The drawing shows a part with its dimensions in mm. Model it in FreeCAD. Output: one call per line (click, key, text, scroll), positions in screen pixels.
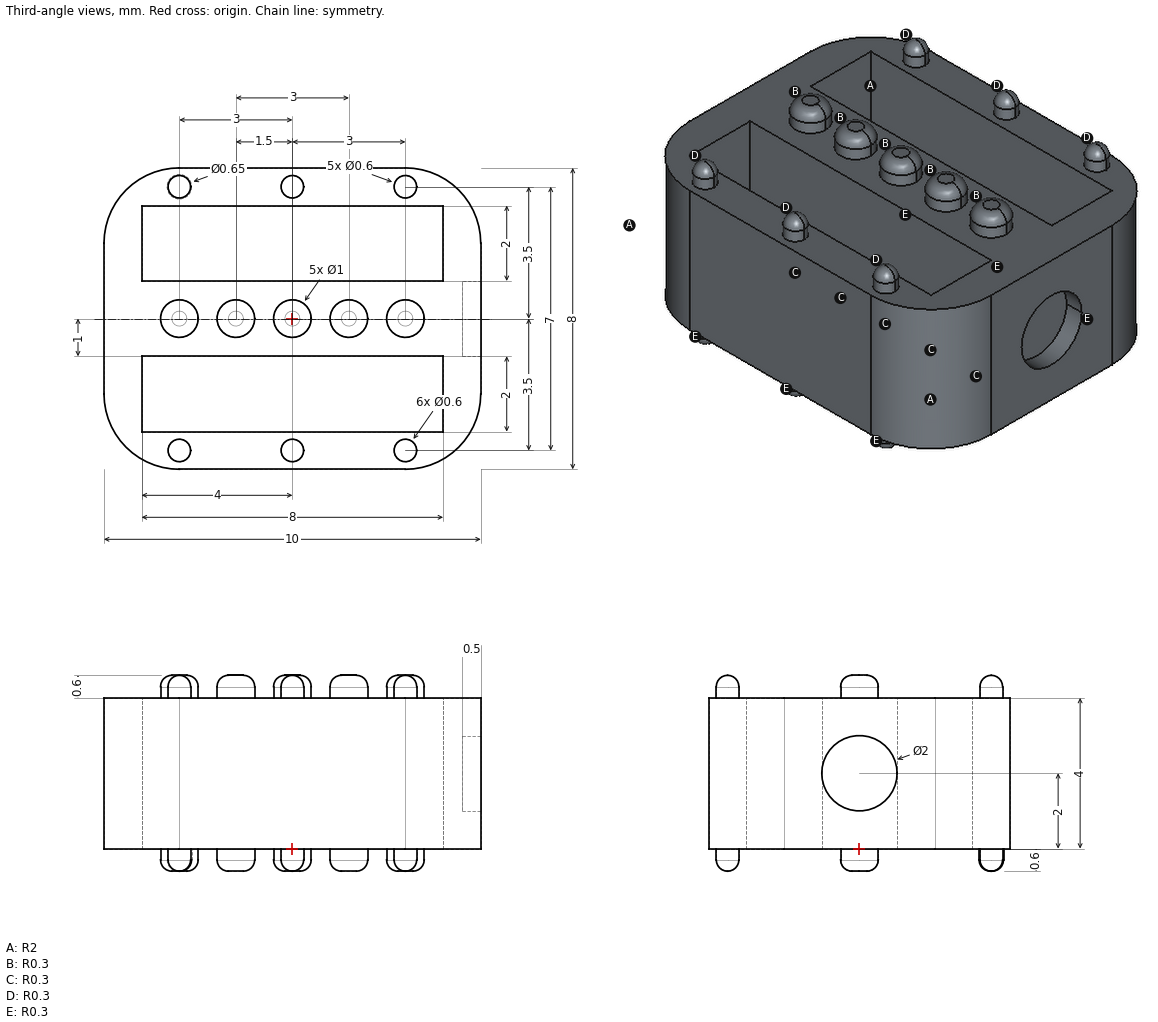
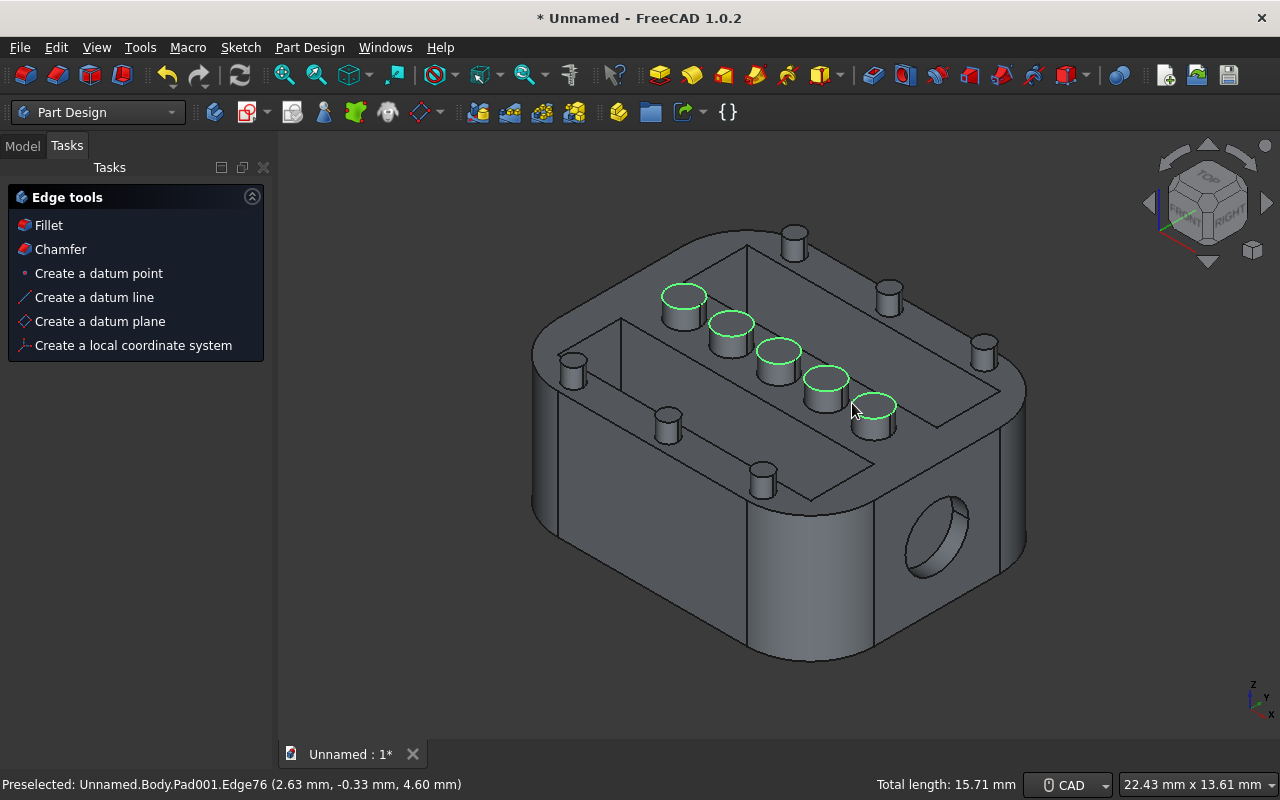
click(26, 76)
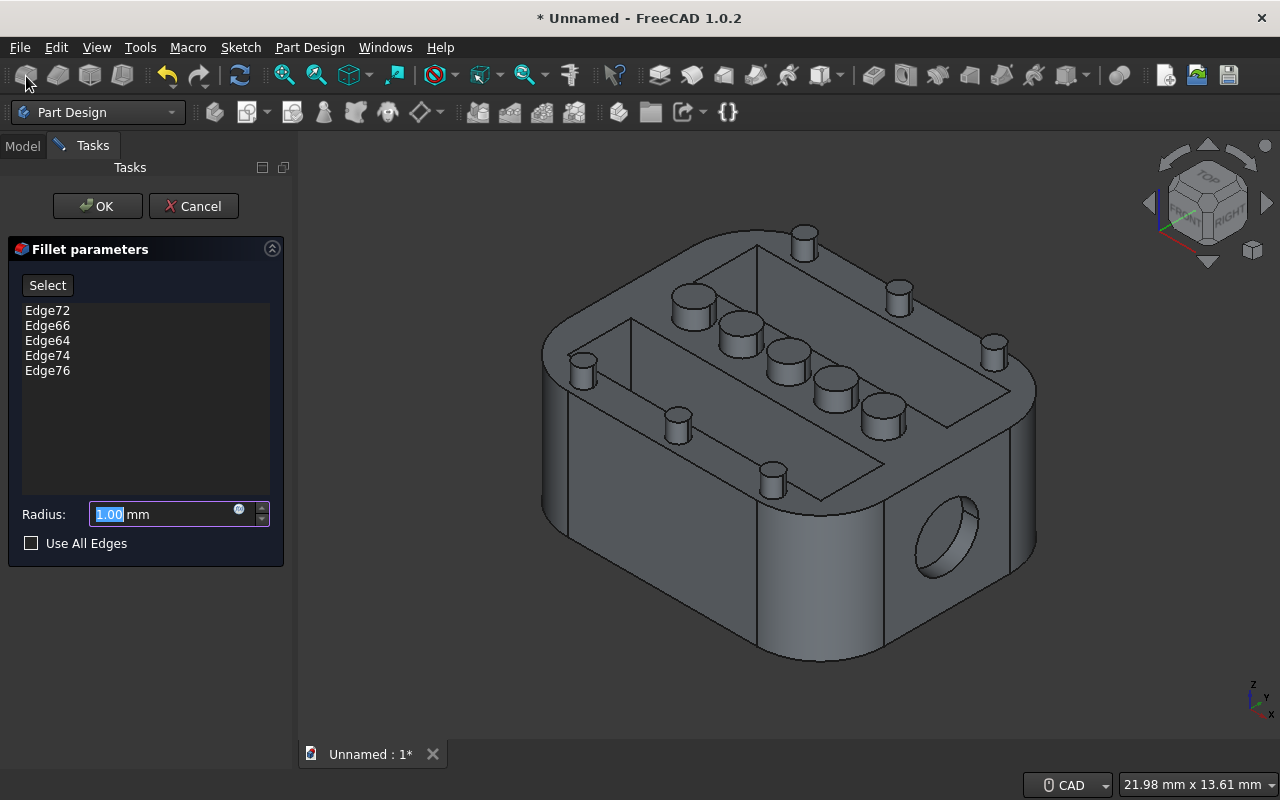
text(0.3)
key(Tab)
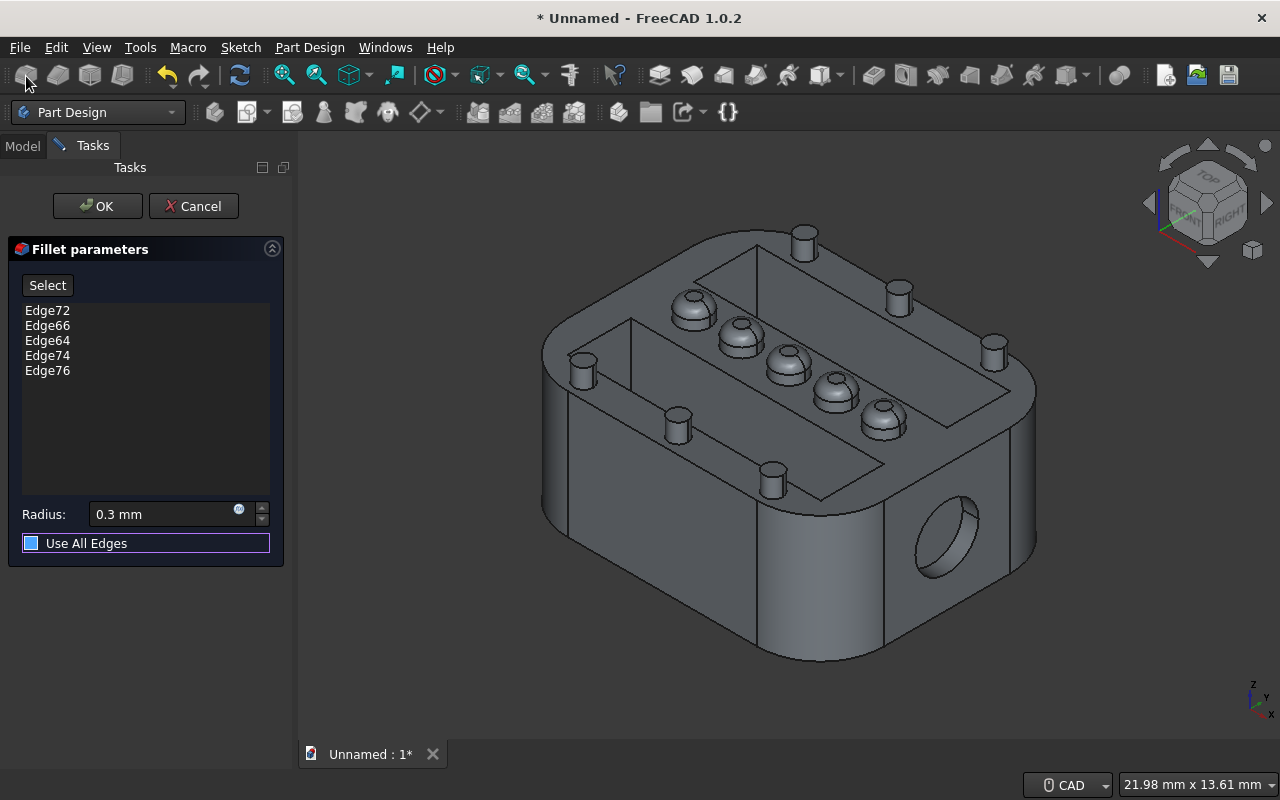
click(98, 206)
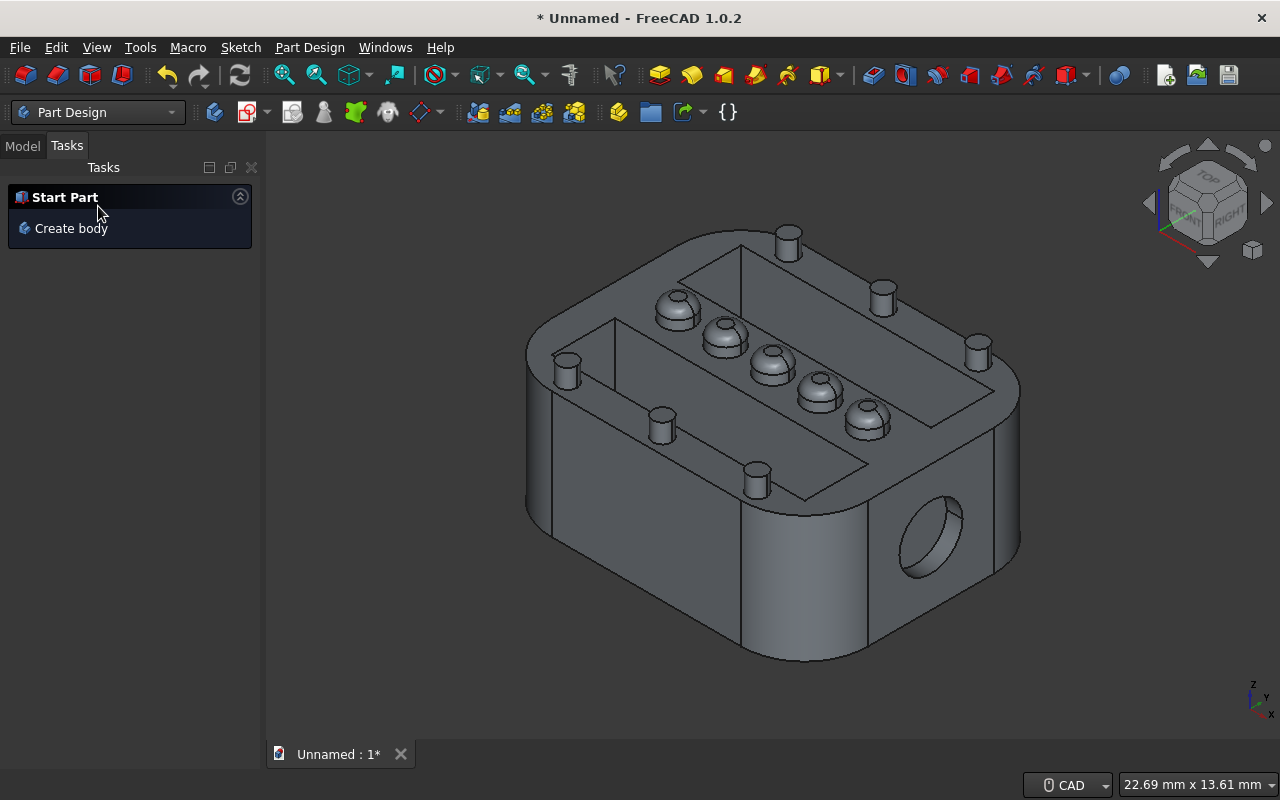
click(23, 145)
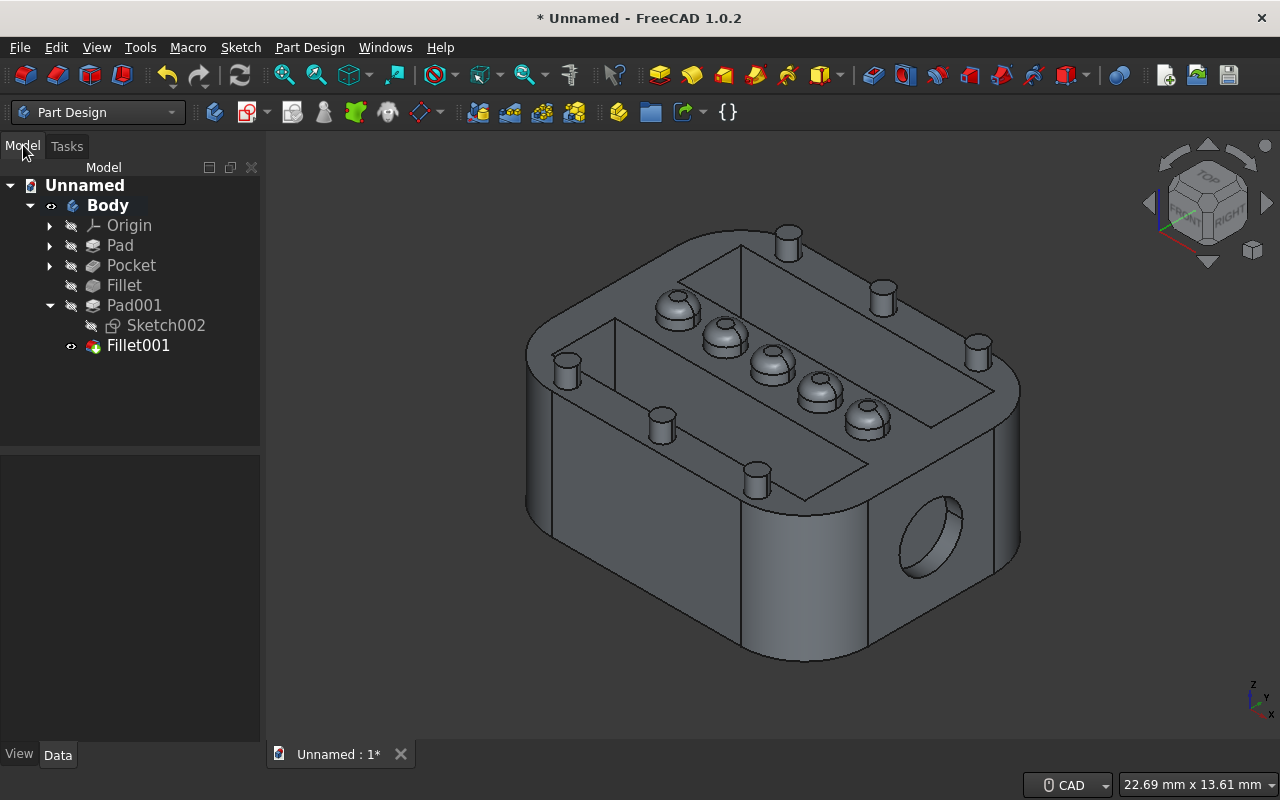
click(50, 226)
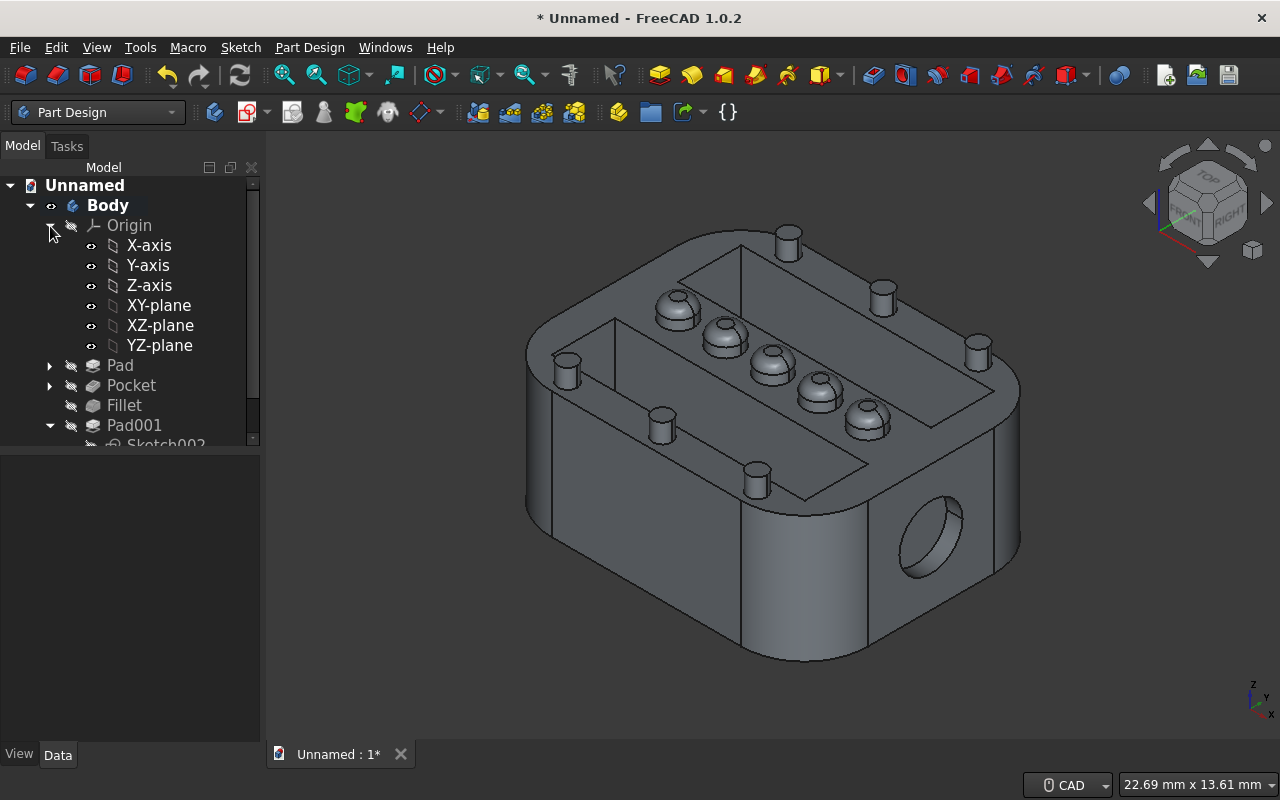
click(136, 306)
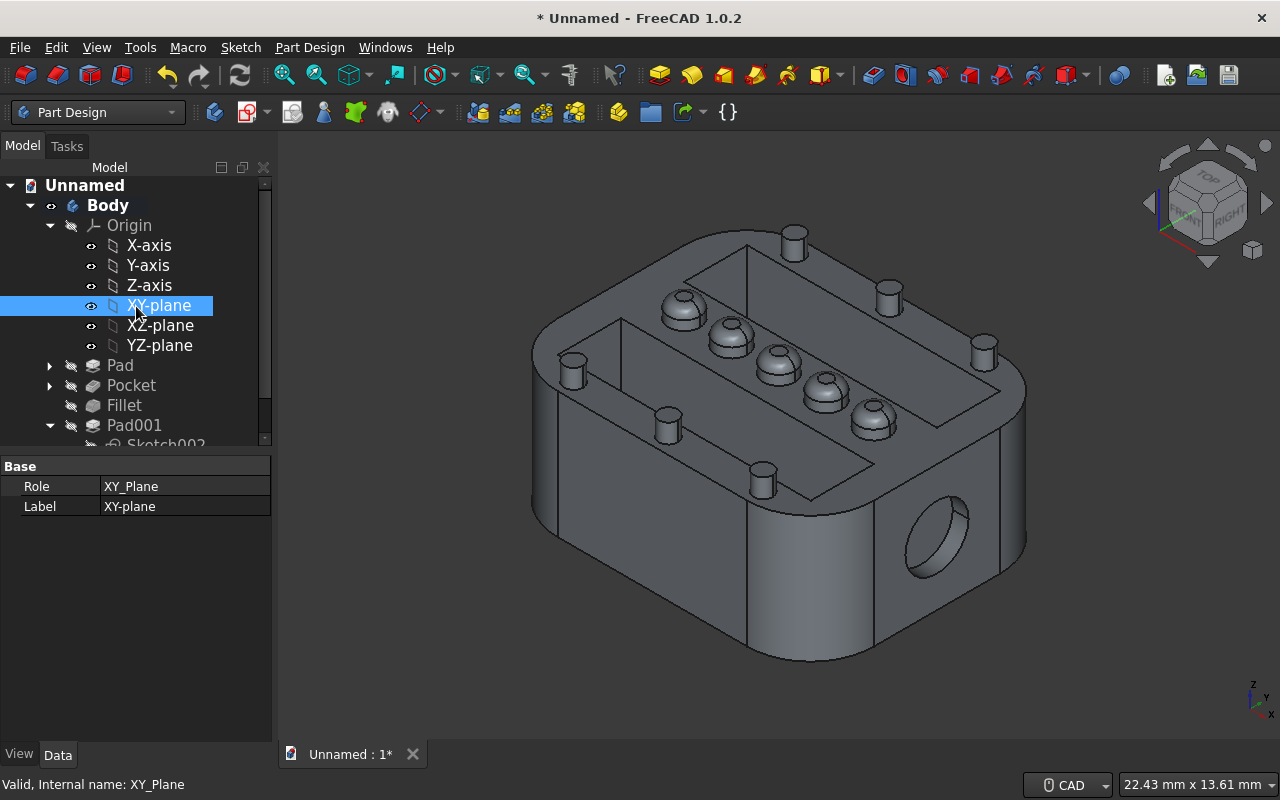
click(420, 112)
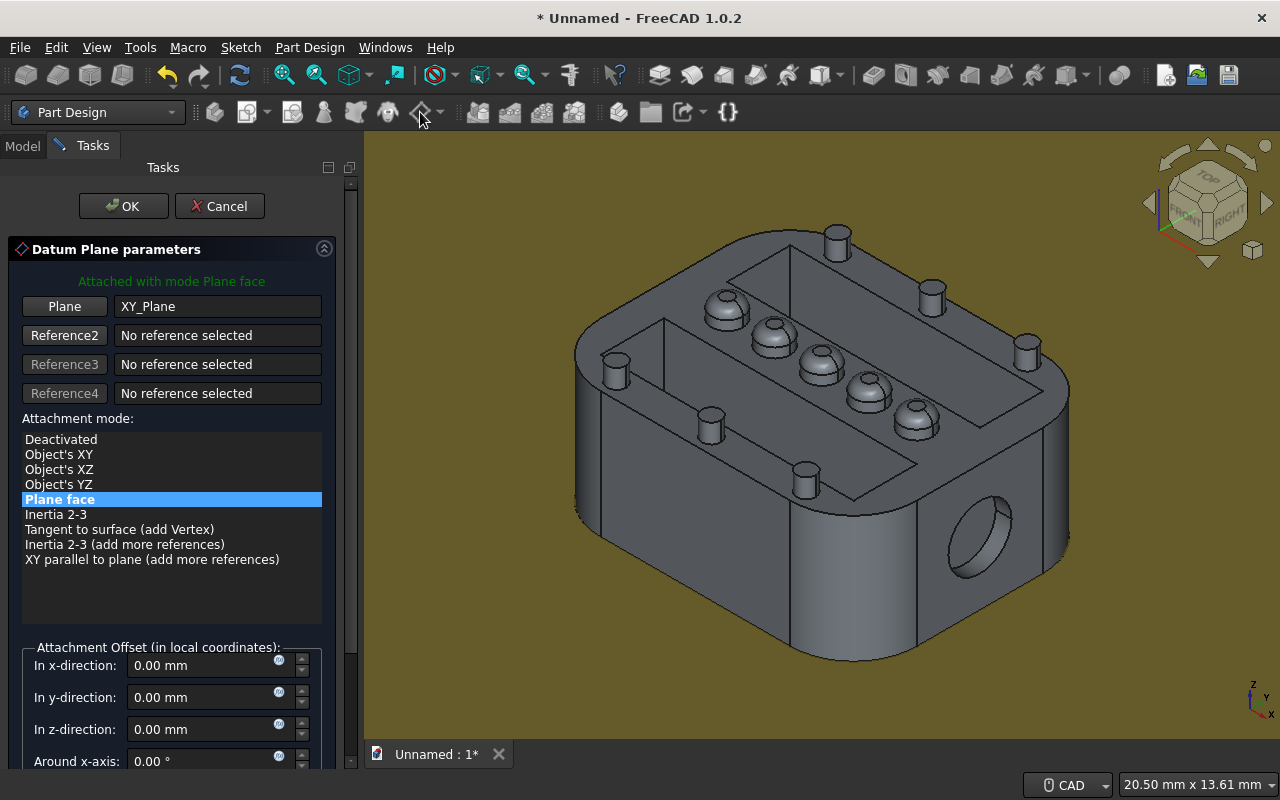
triple_click(210, 729)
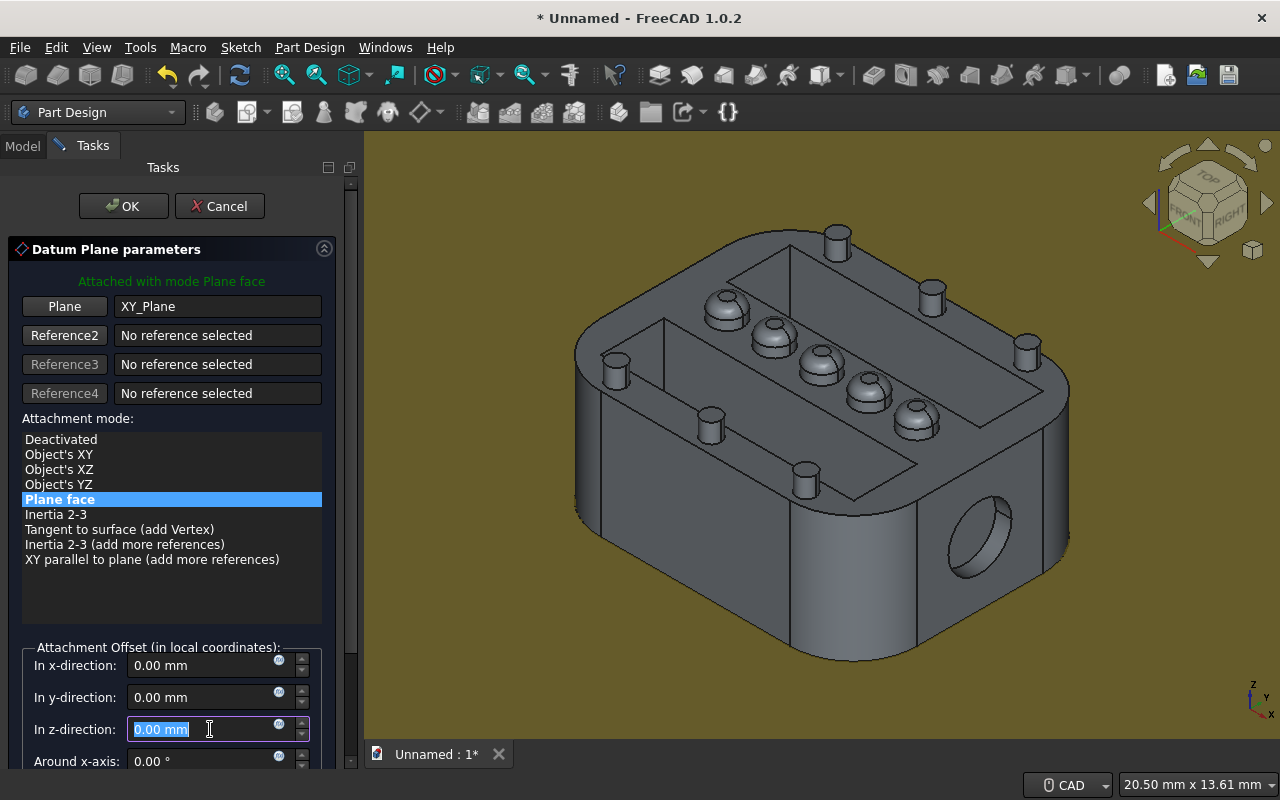
text(-0.6)
key(Tab)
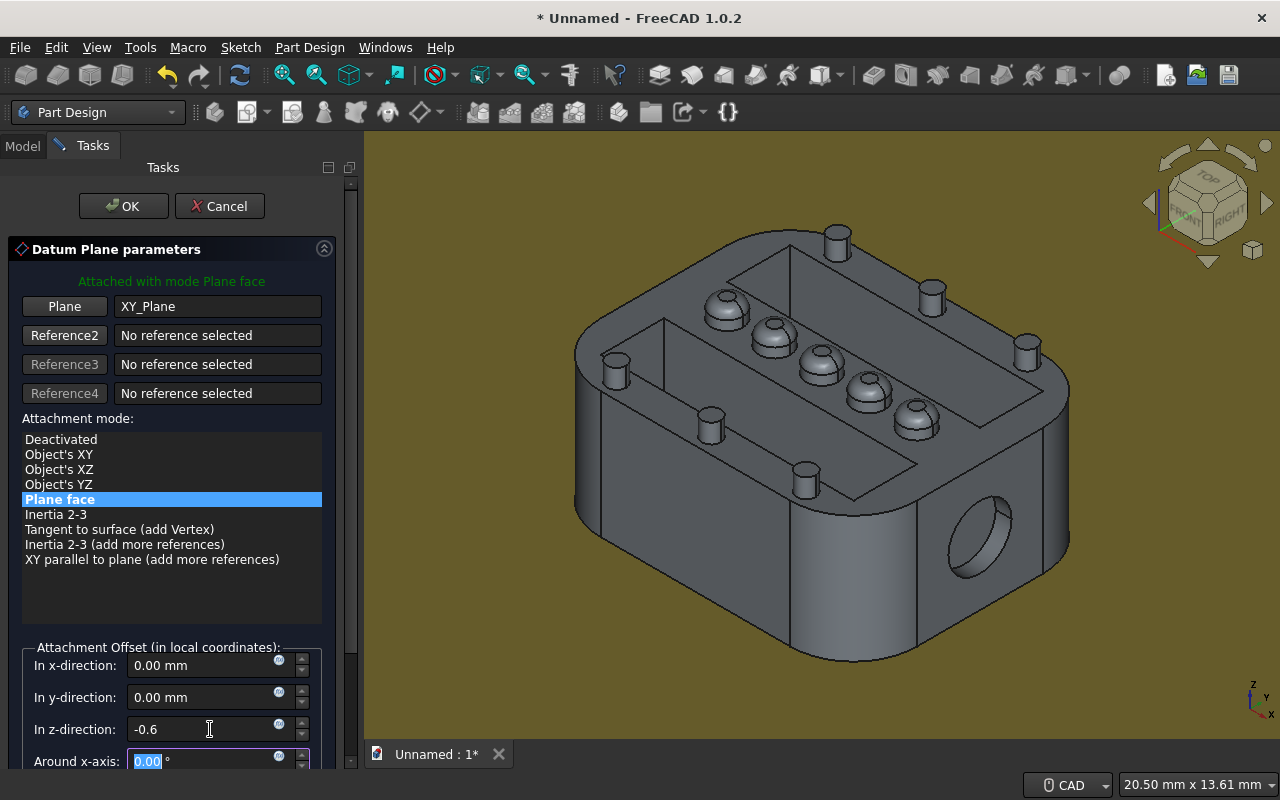
click(124, 206)